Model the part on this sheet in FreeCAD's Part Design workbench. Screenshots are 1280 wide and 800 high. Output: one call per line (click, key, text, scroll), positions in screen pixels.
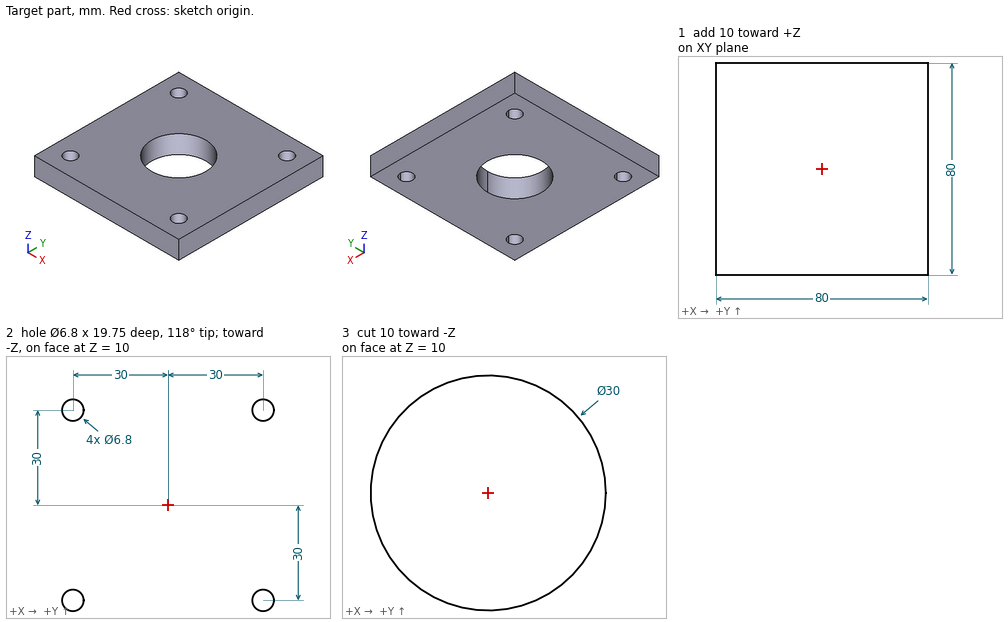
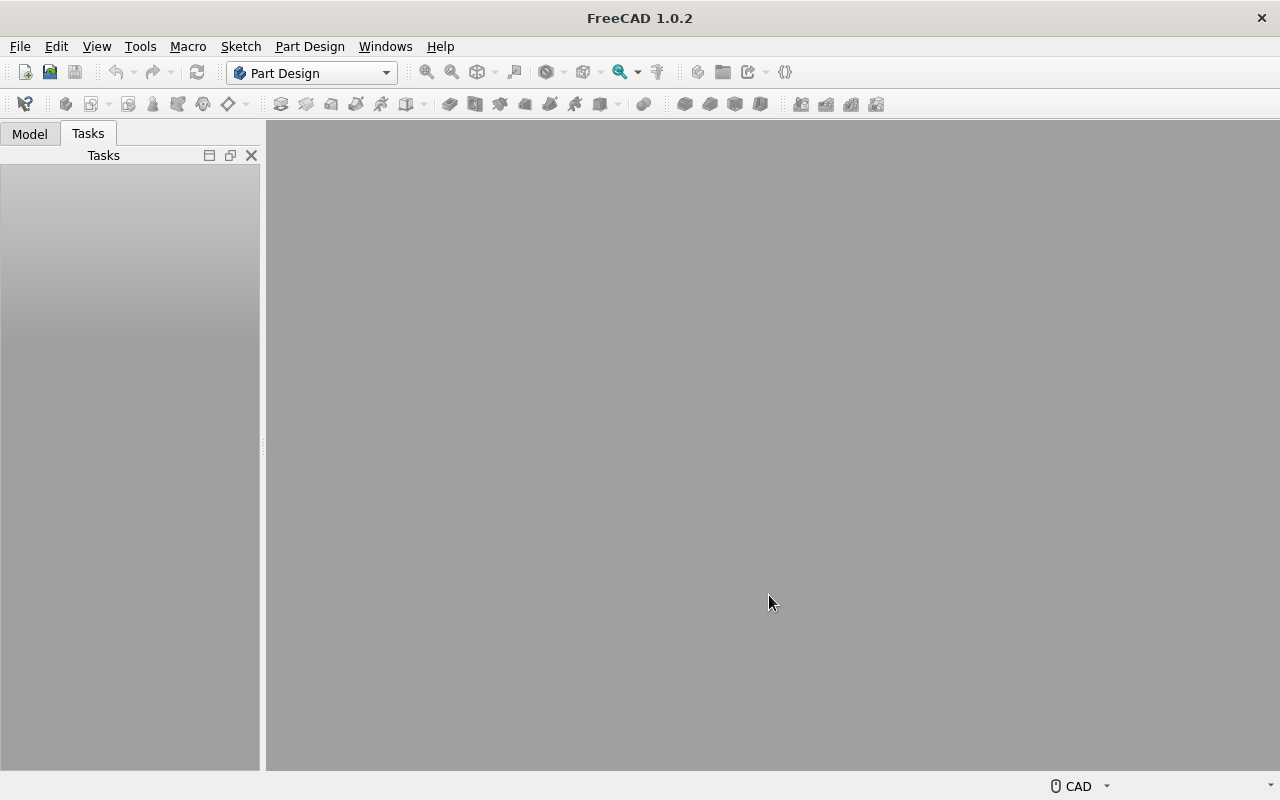
key(ctrl+n)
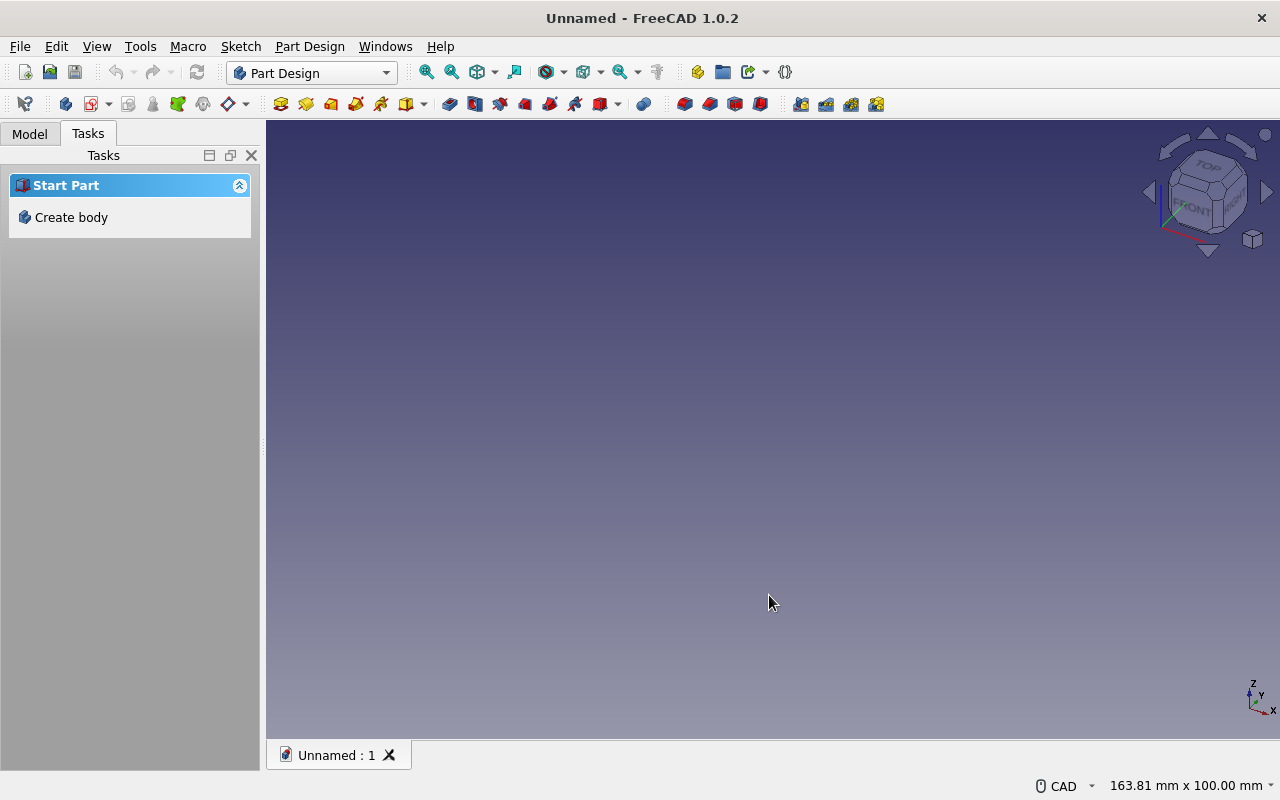
click(90, 104)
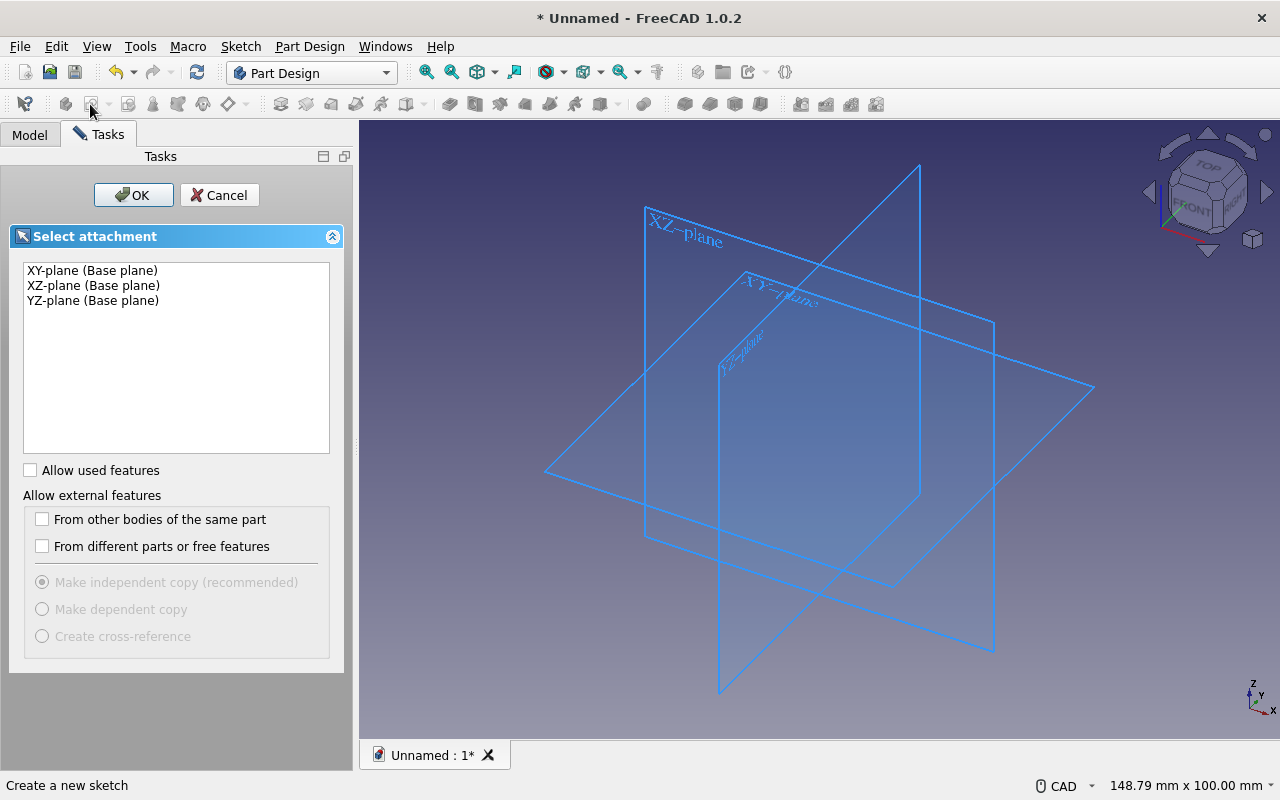
click(84, 270)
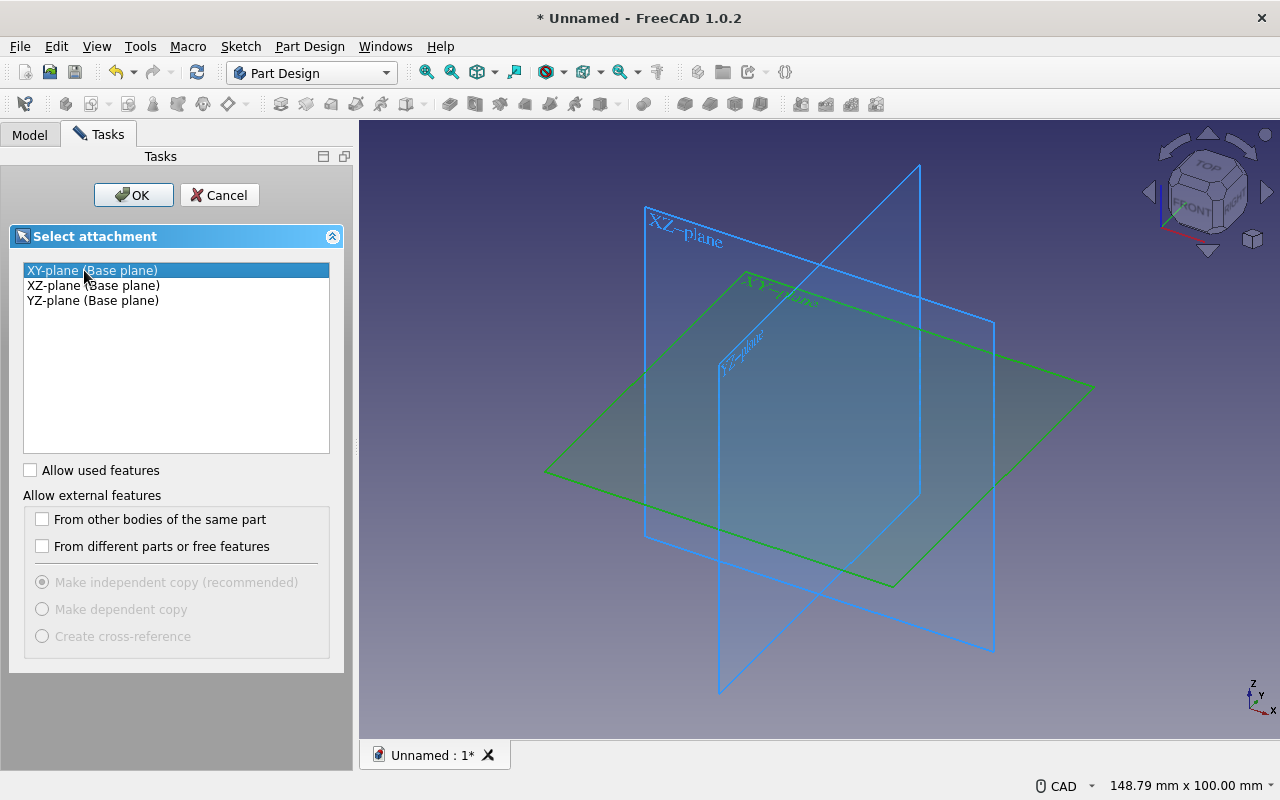
click(134, 195)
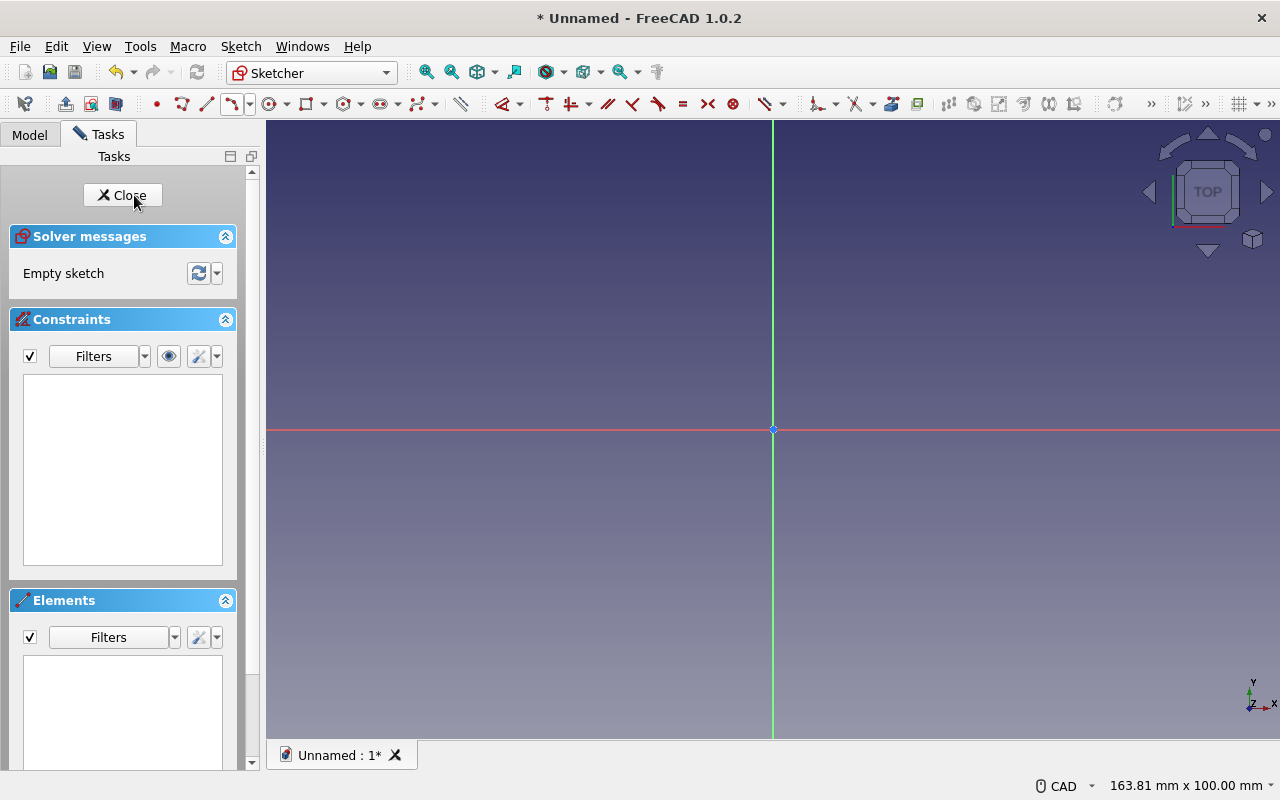
key(g)
key(v)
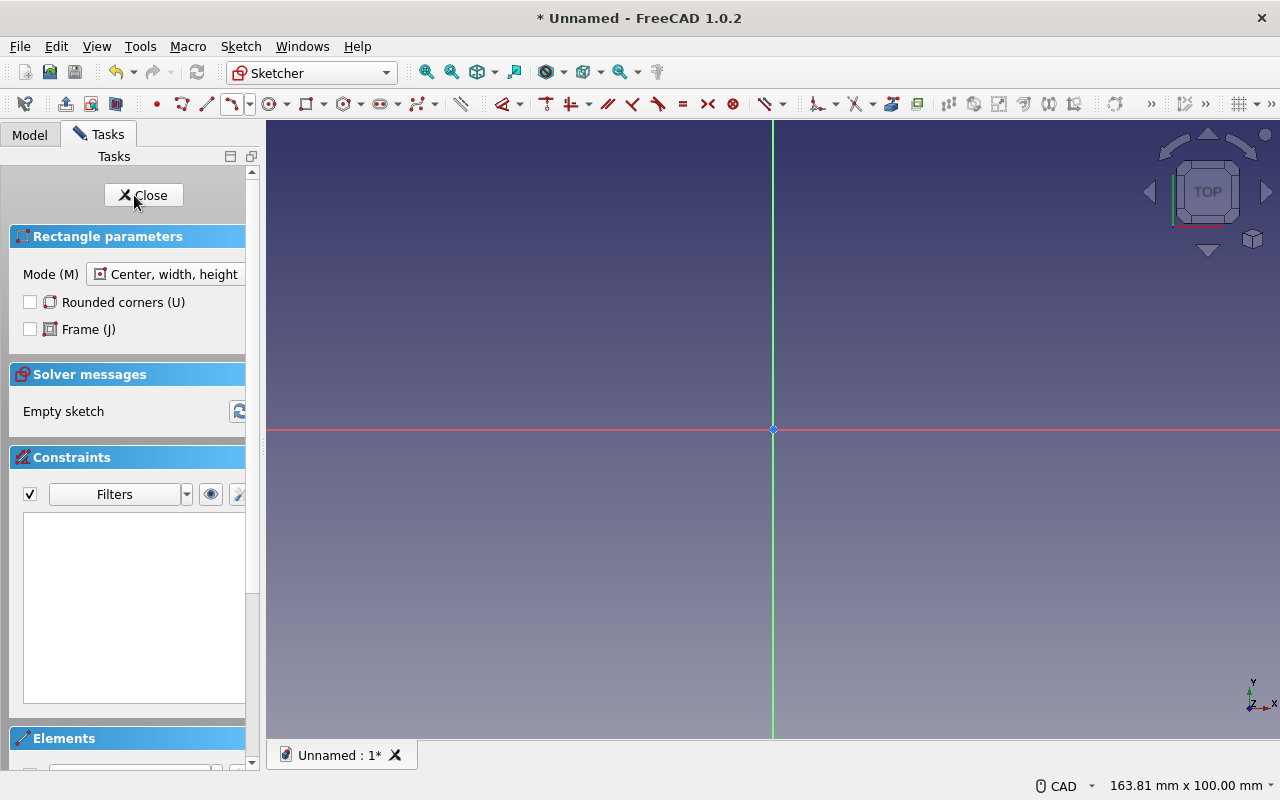
click(773, 430)
move(1021, 182)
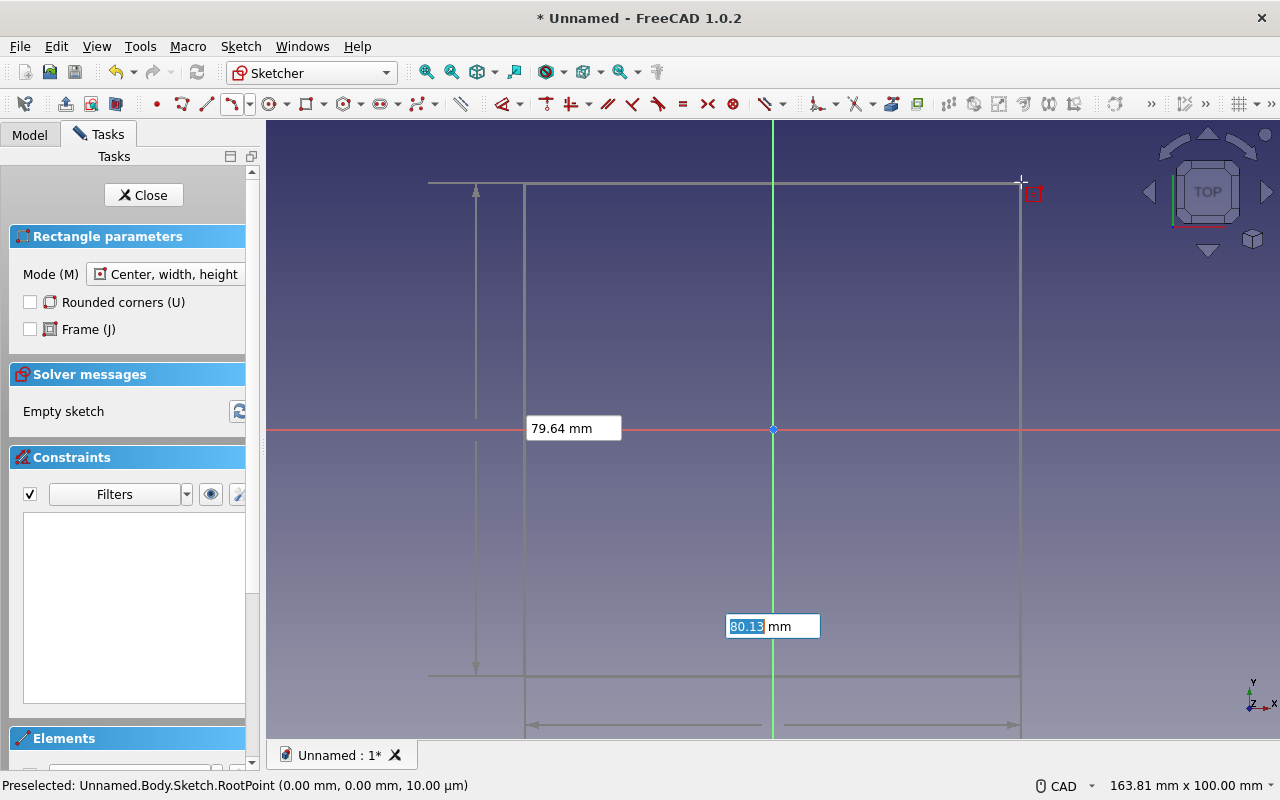
text(80)
key(Tab)
text(80)
key(Return)
key(Escape)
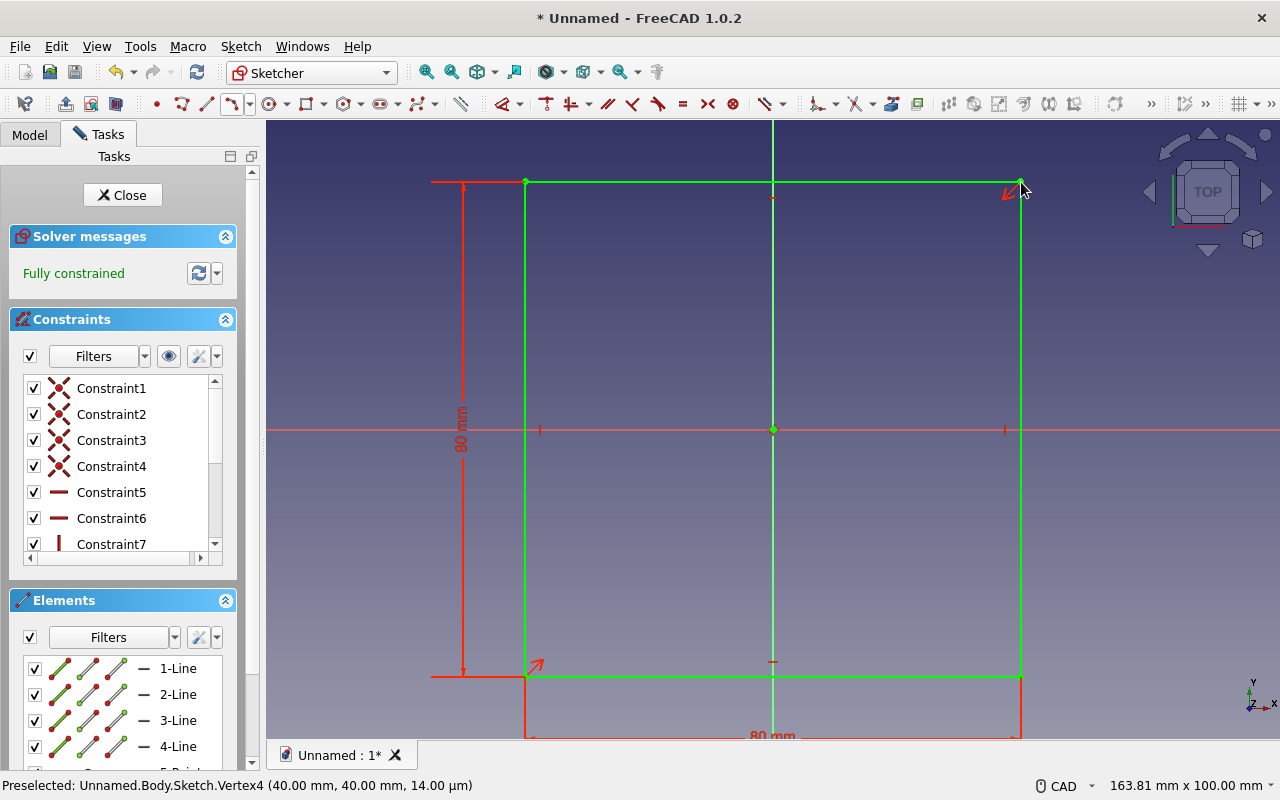
click(123, 195)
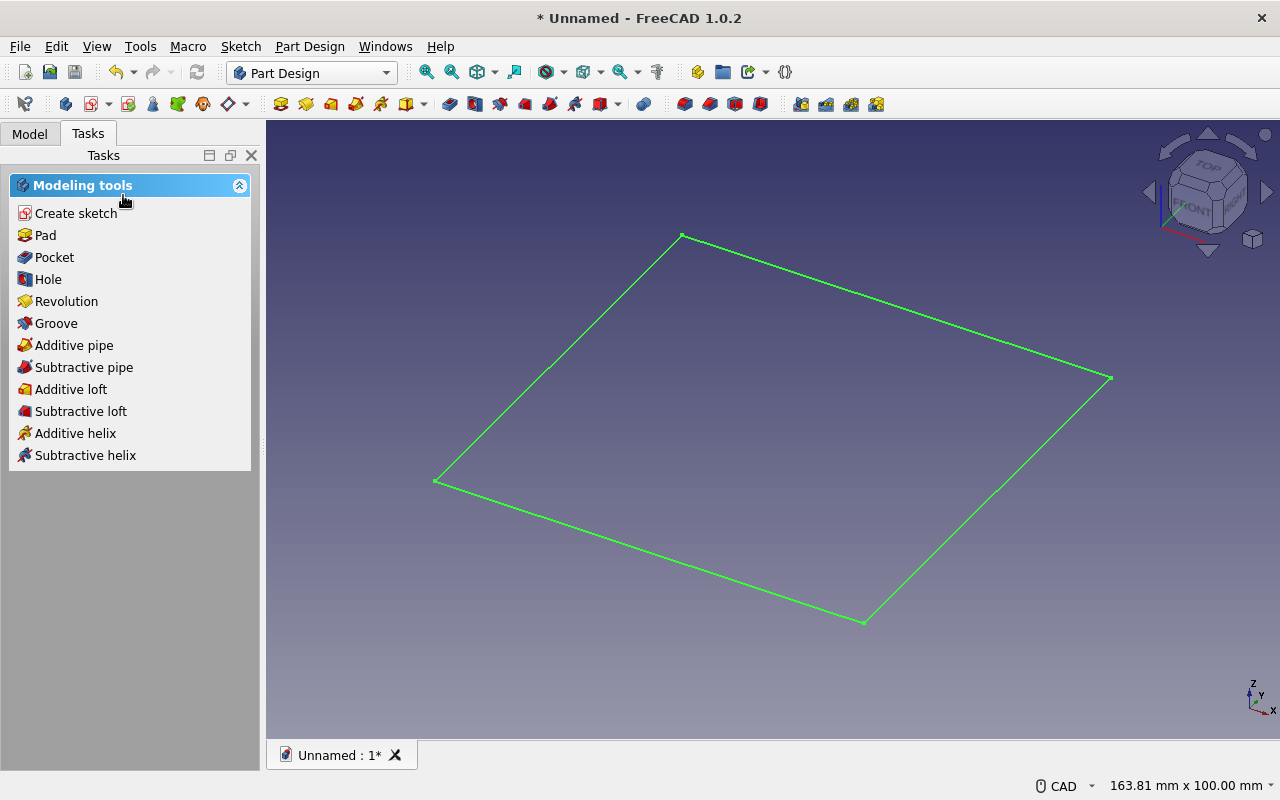
click(281, 104)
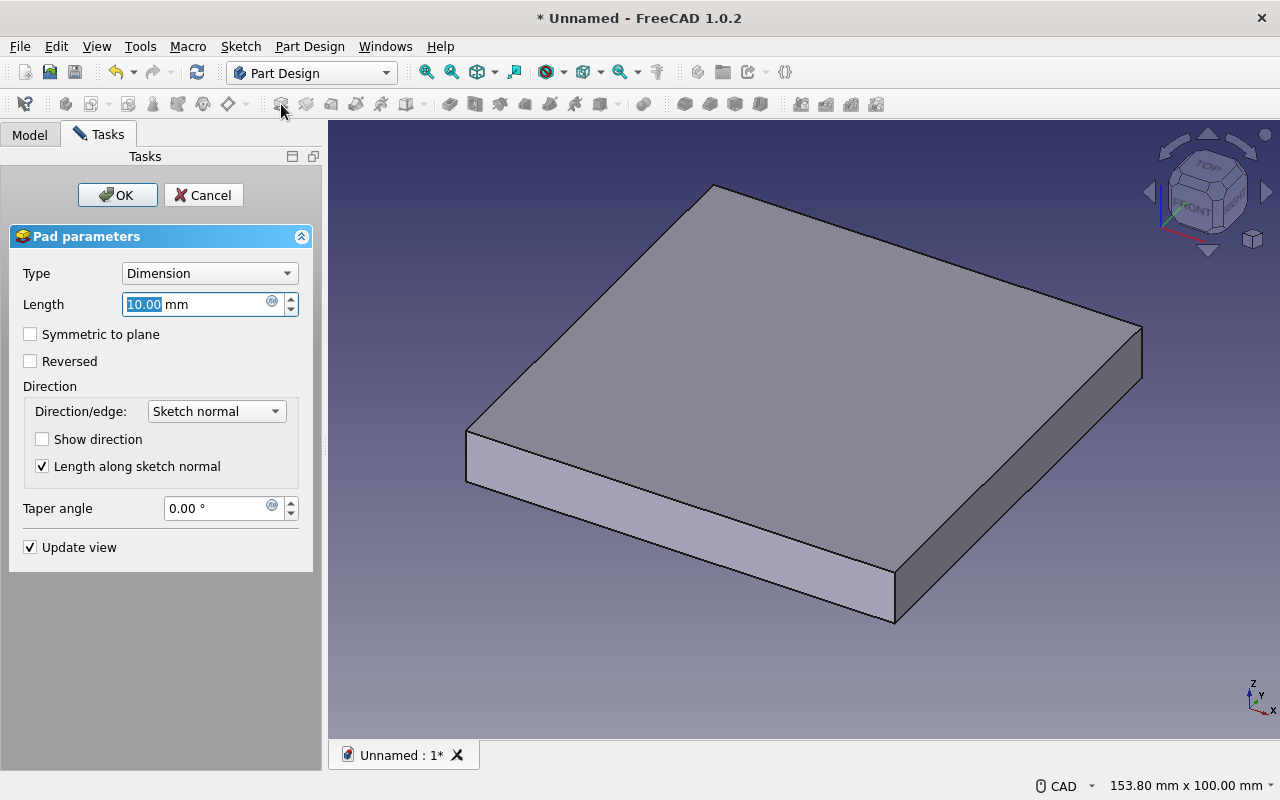
text(10)
key(Tab)